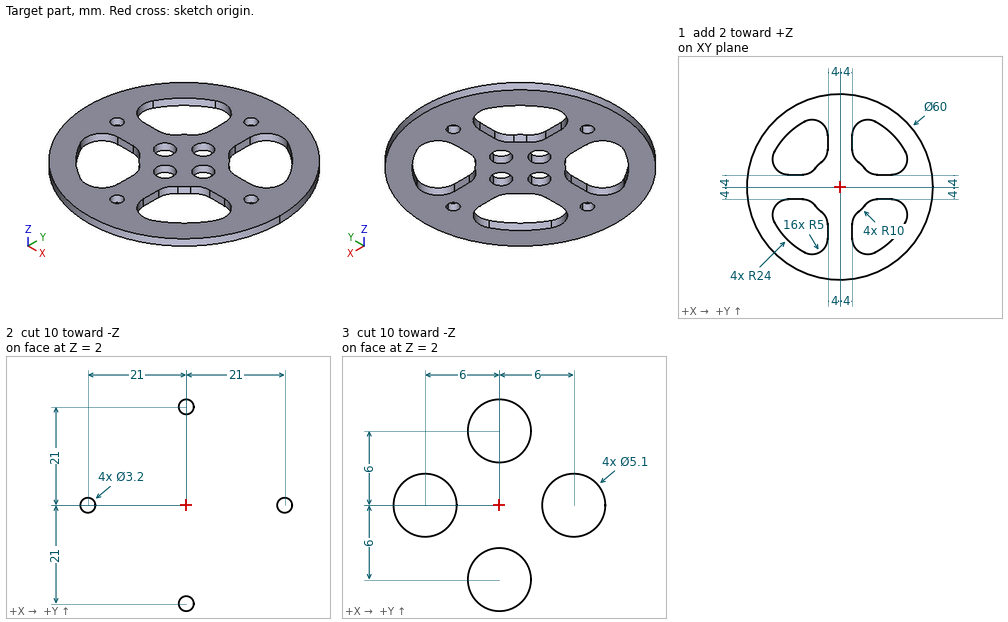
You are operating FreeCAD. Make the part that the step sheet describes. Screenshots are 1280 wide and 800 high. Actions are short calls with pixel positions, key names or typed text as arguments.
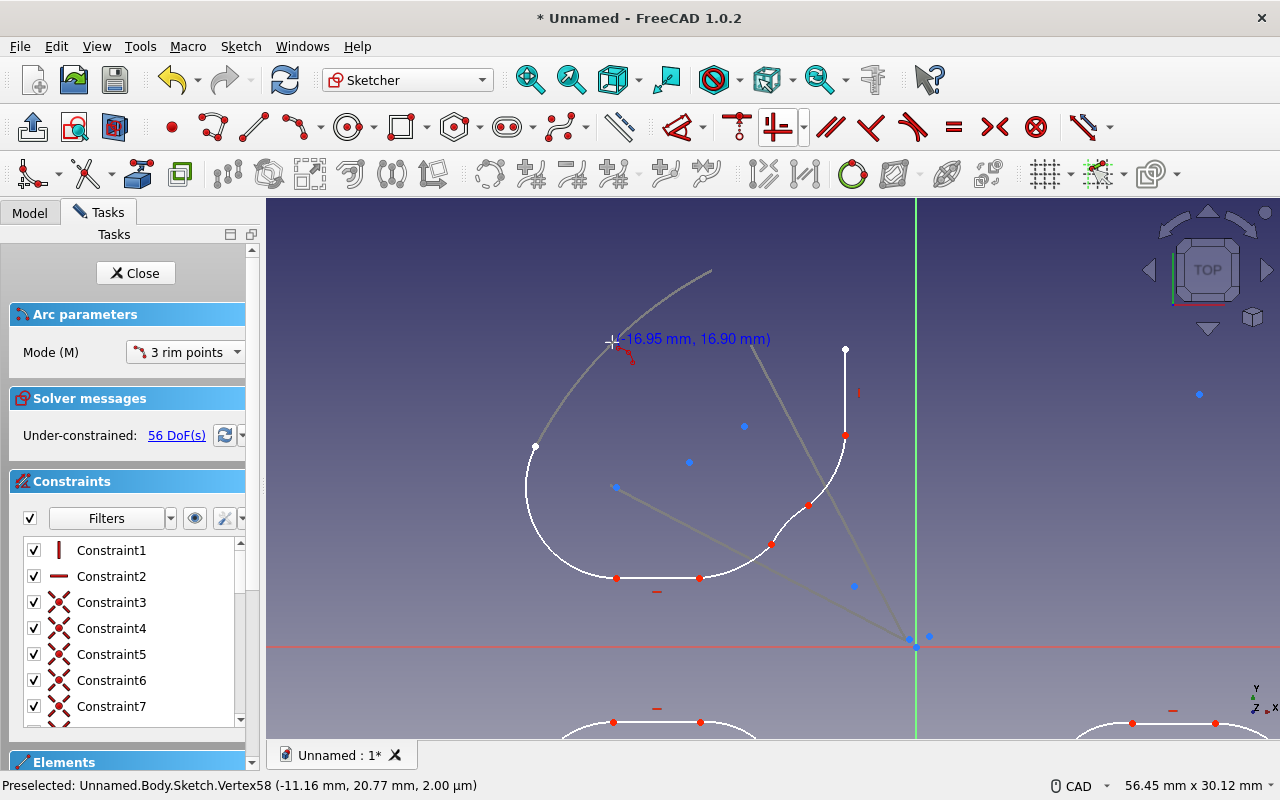
click(611, 343)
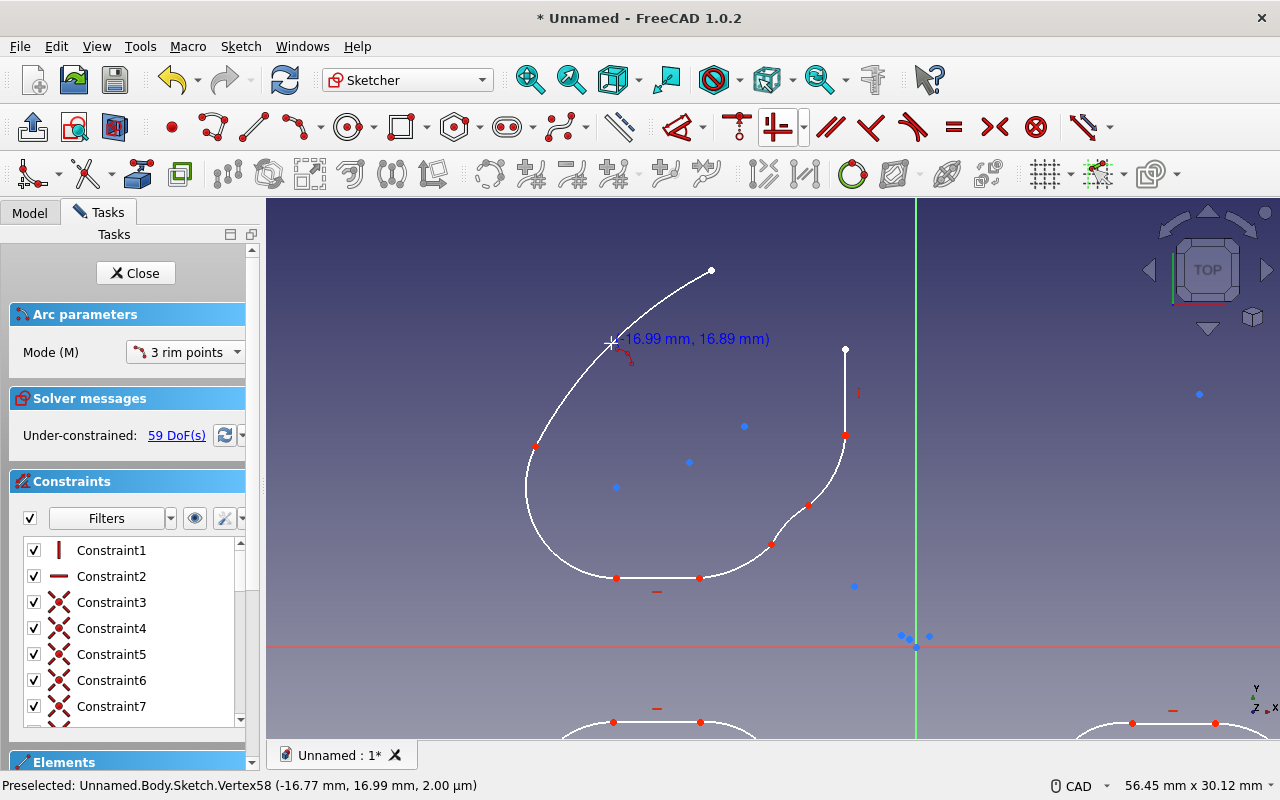
click(712, 270)
click(845, 349)
click(801, 270)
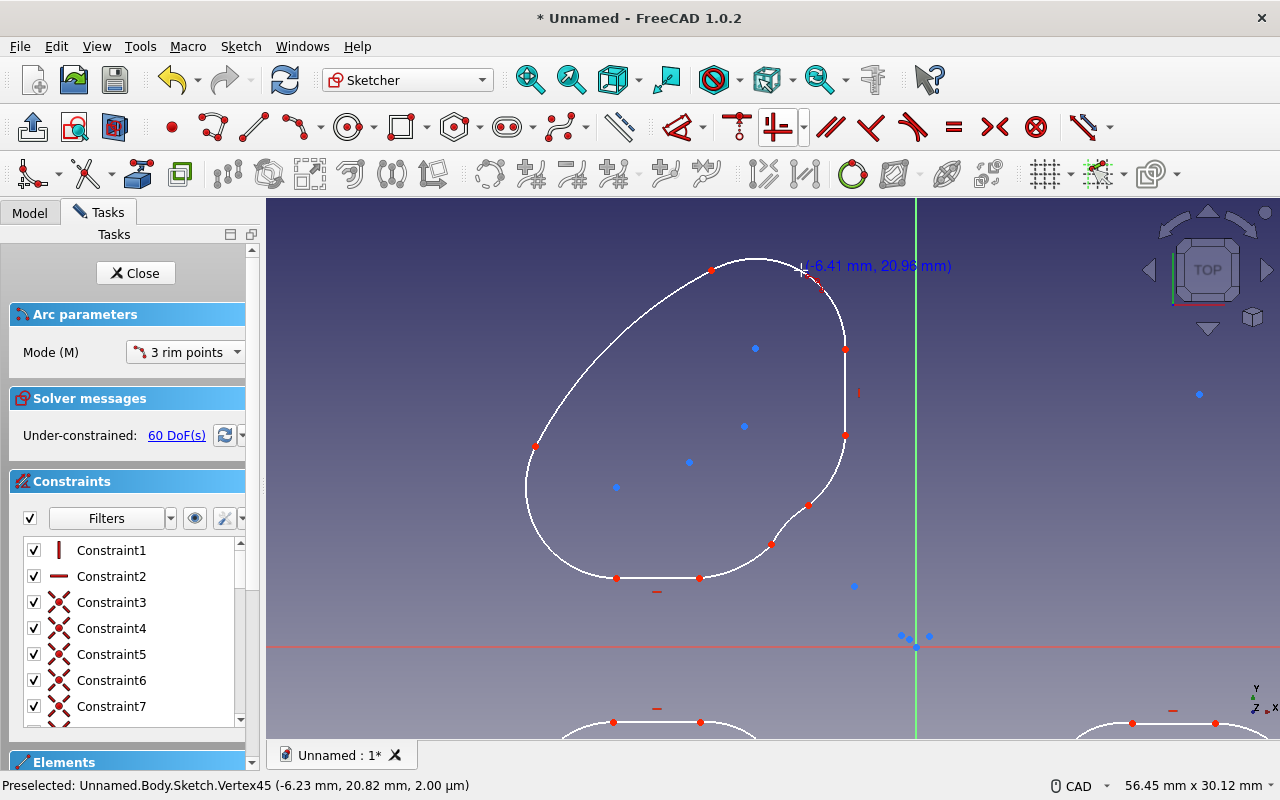
key(g)
key(l)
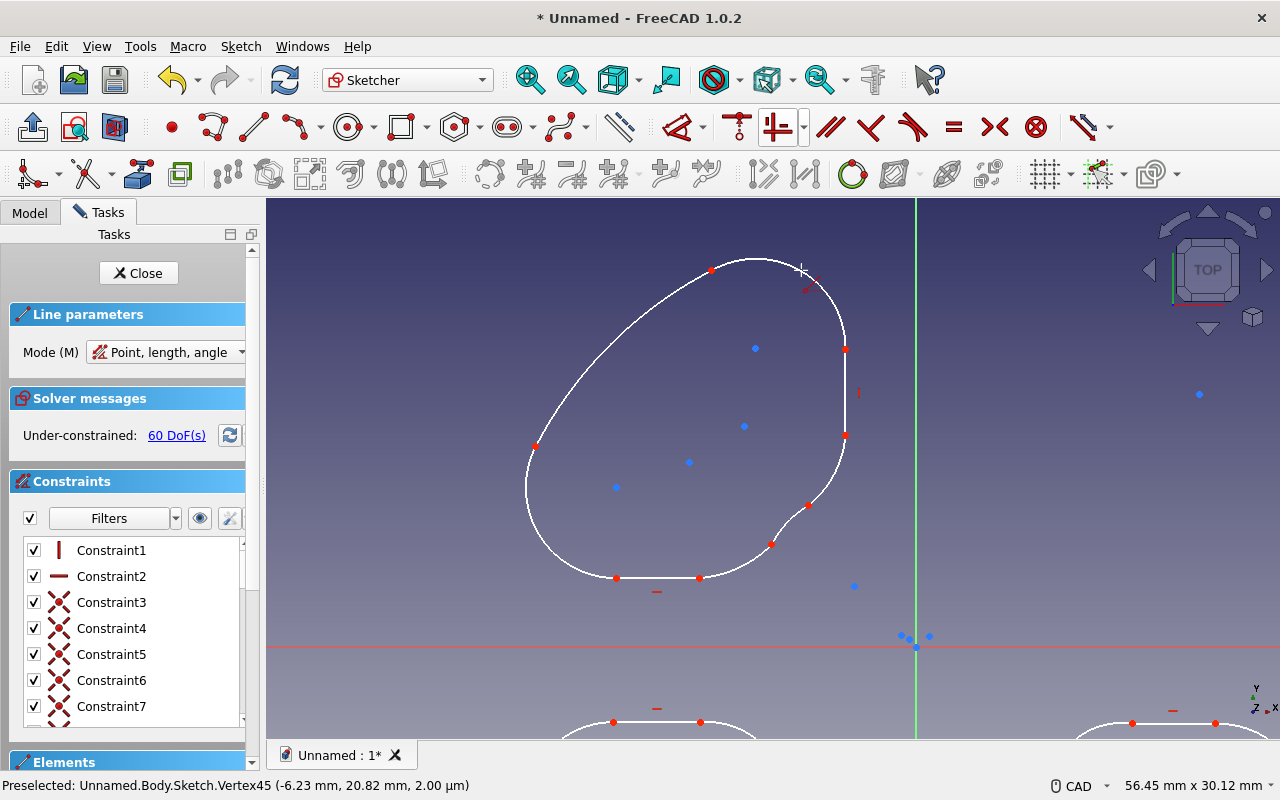
click(988, 432)
click(988, 347)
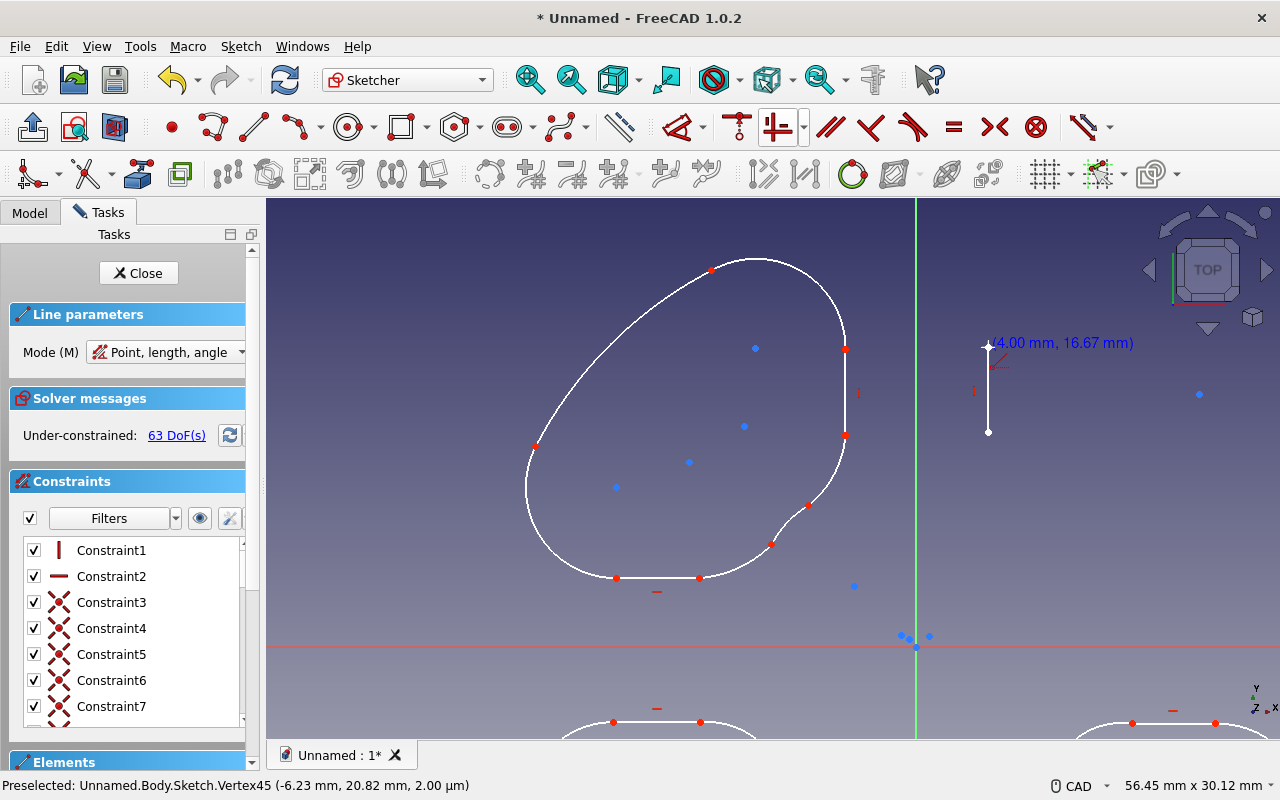
scroll(613, 391, down, 6)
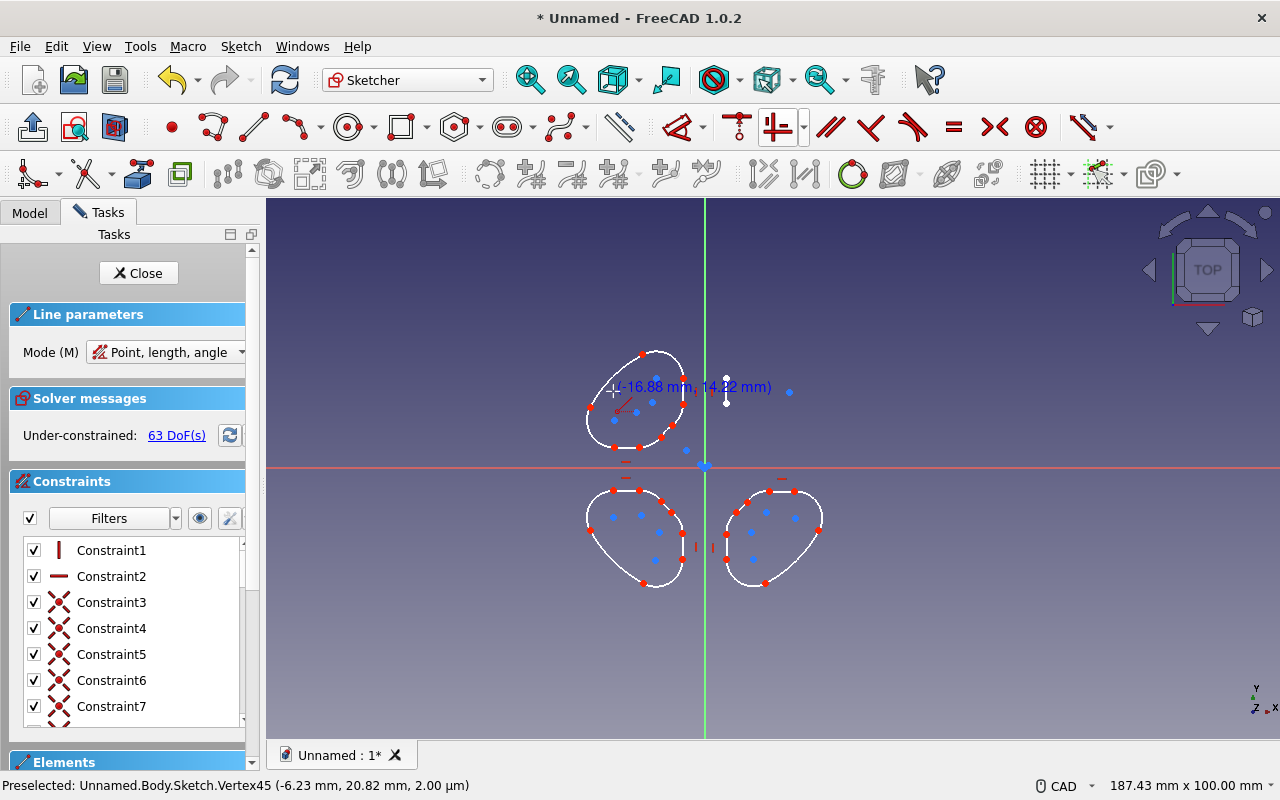
click(795, 447)
click(769, 447)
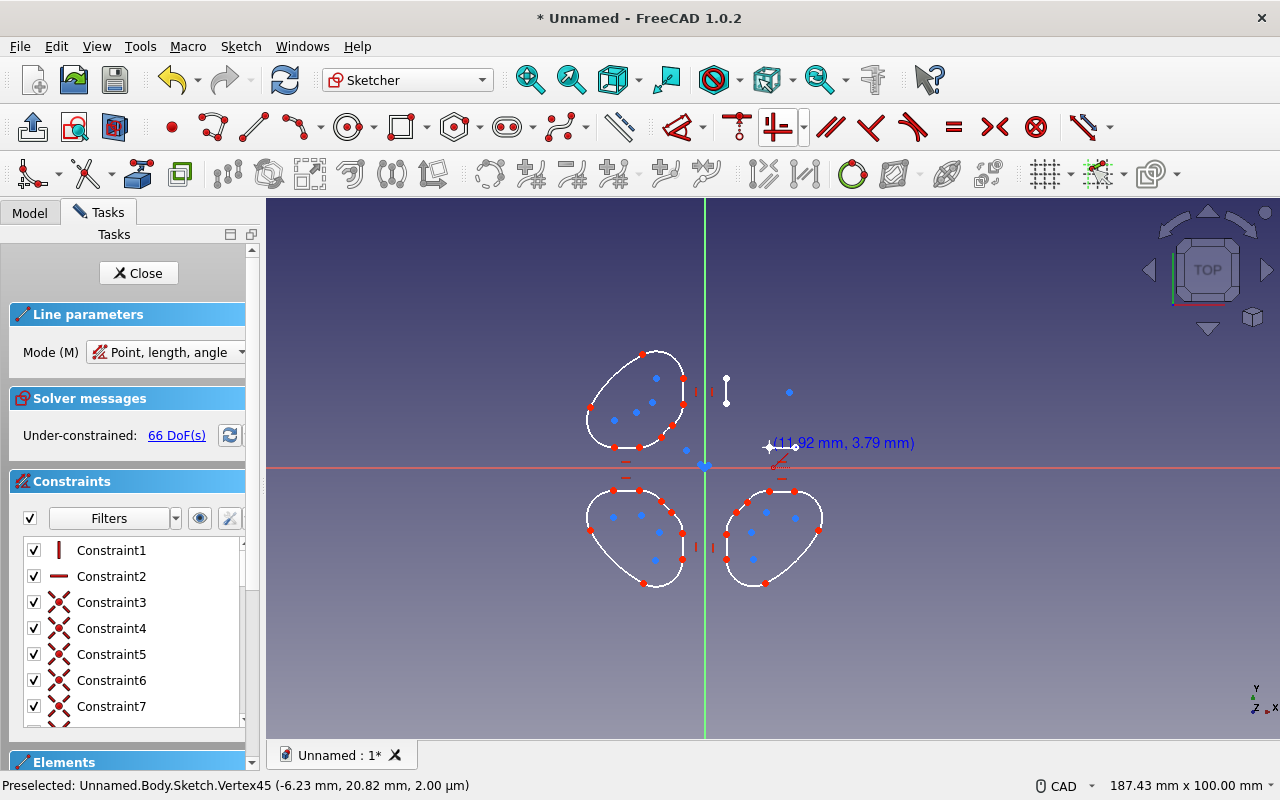
key(g)
key(3)
key(a)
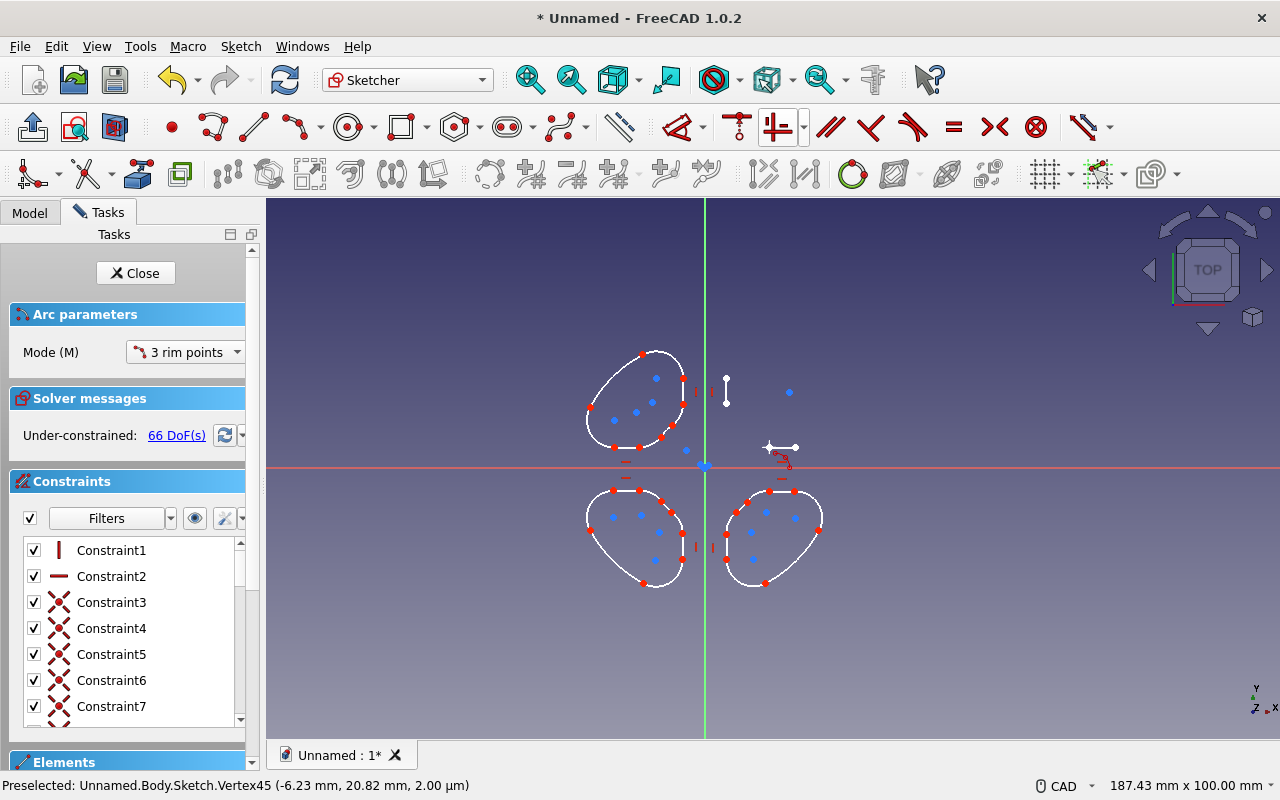
scroll(726, 378, up, 2)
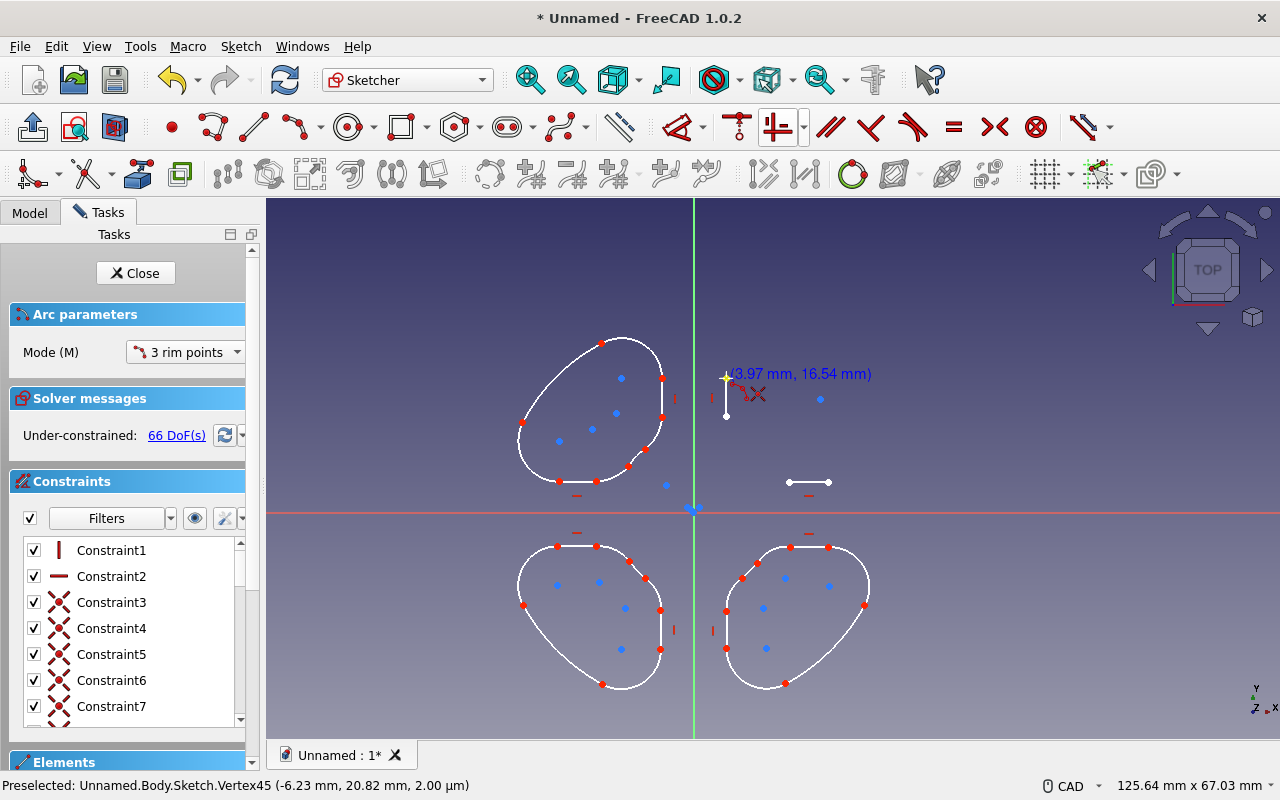
click(726, 378)
click(786, 342)
click(746, 343)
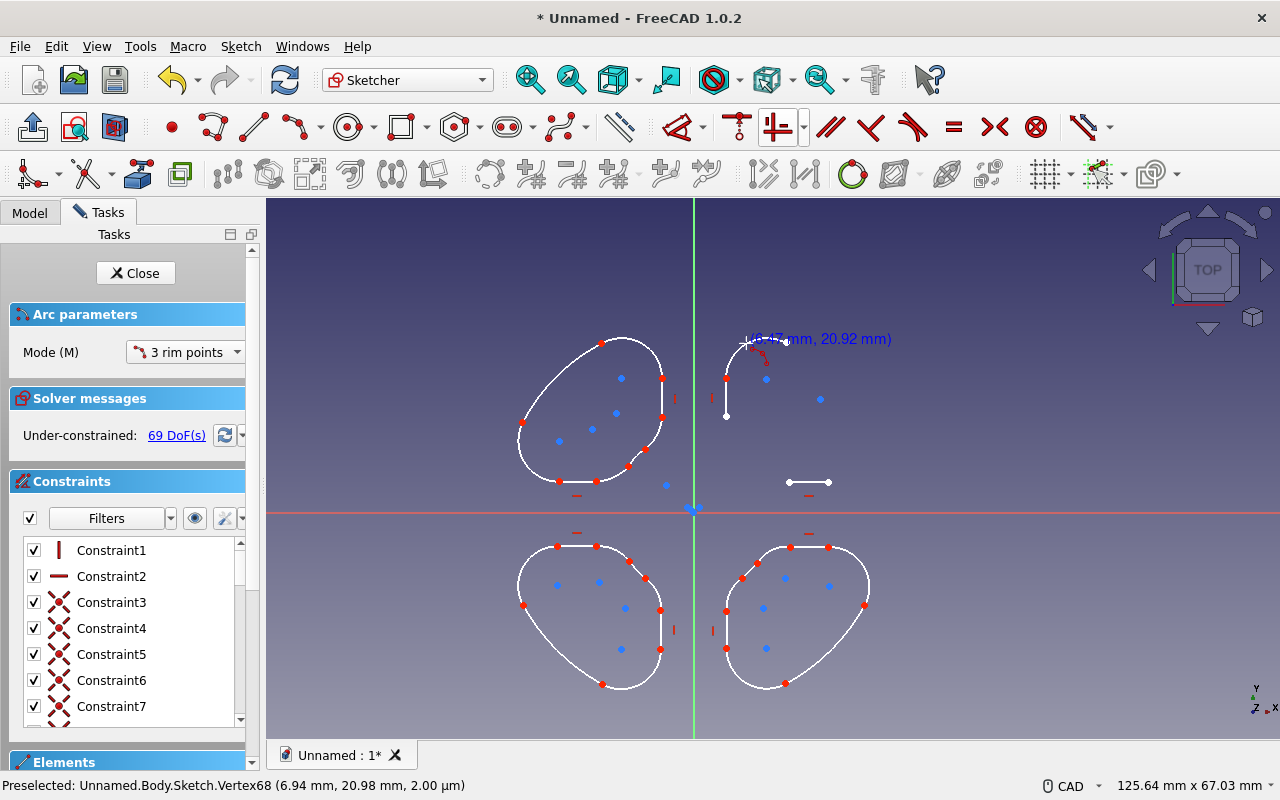
click(786, 343)
click(864, 421)